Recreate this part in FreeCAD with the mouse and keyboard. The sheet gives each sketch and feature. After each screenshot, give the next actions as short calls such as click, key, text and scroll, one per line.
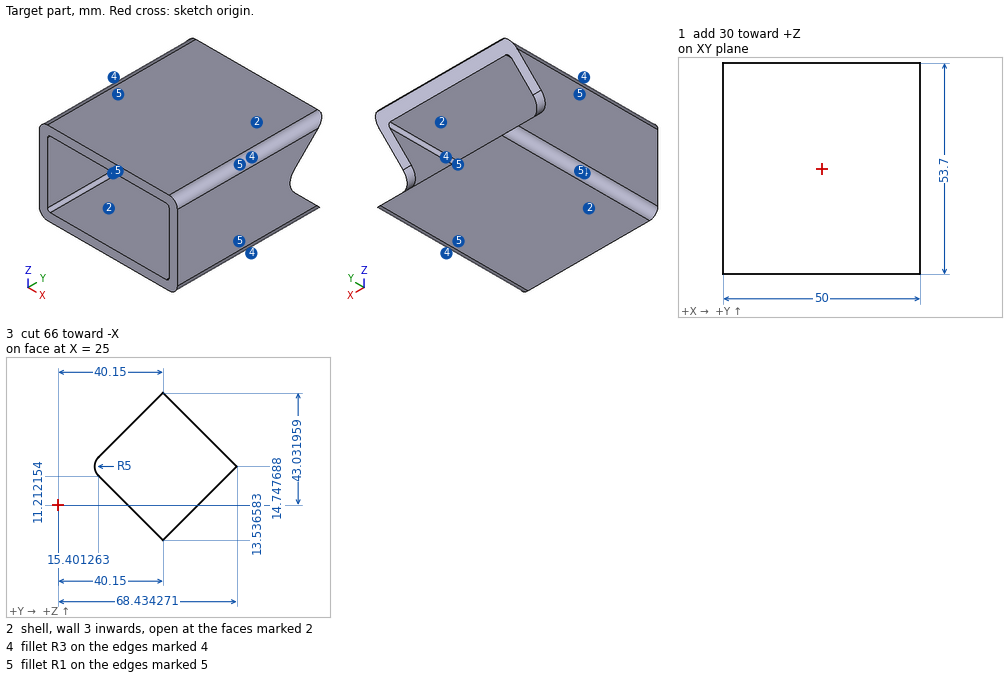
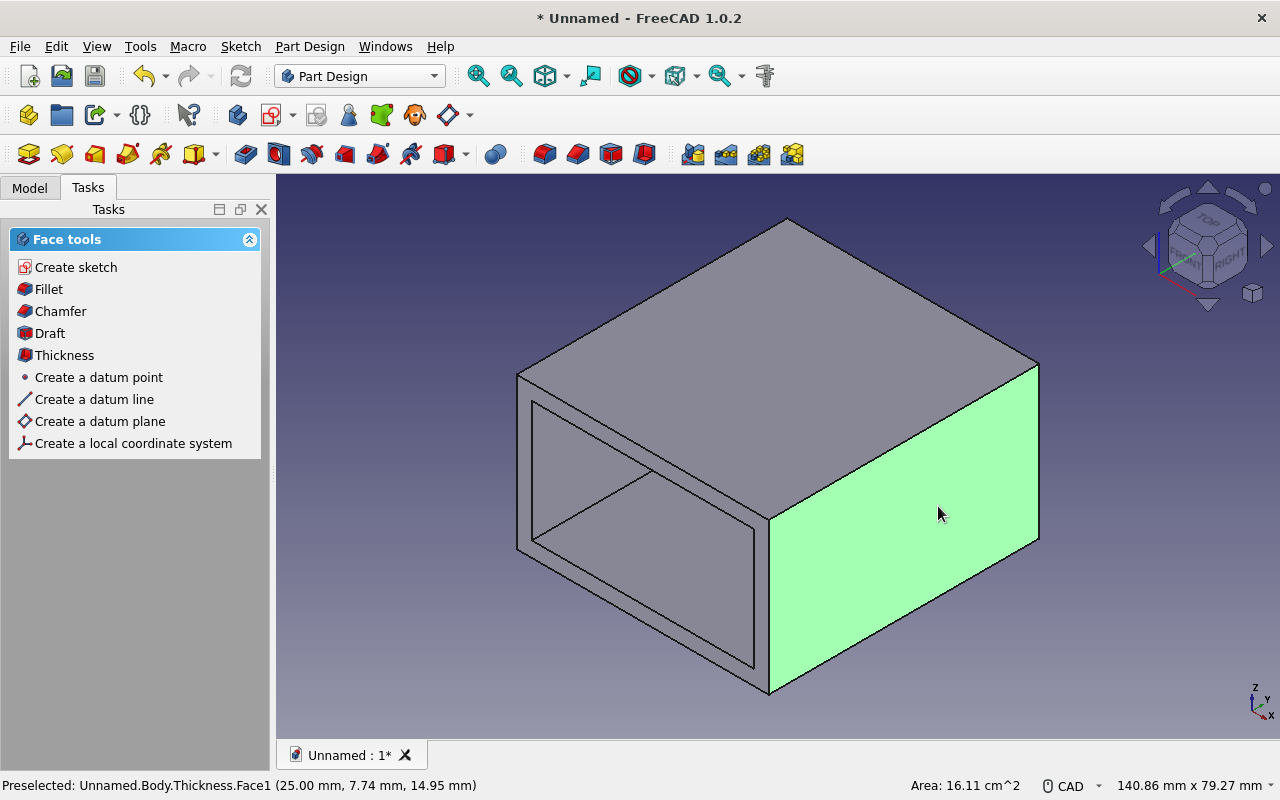
click(270, 116)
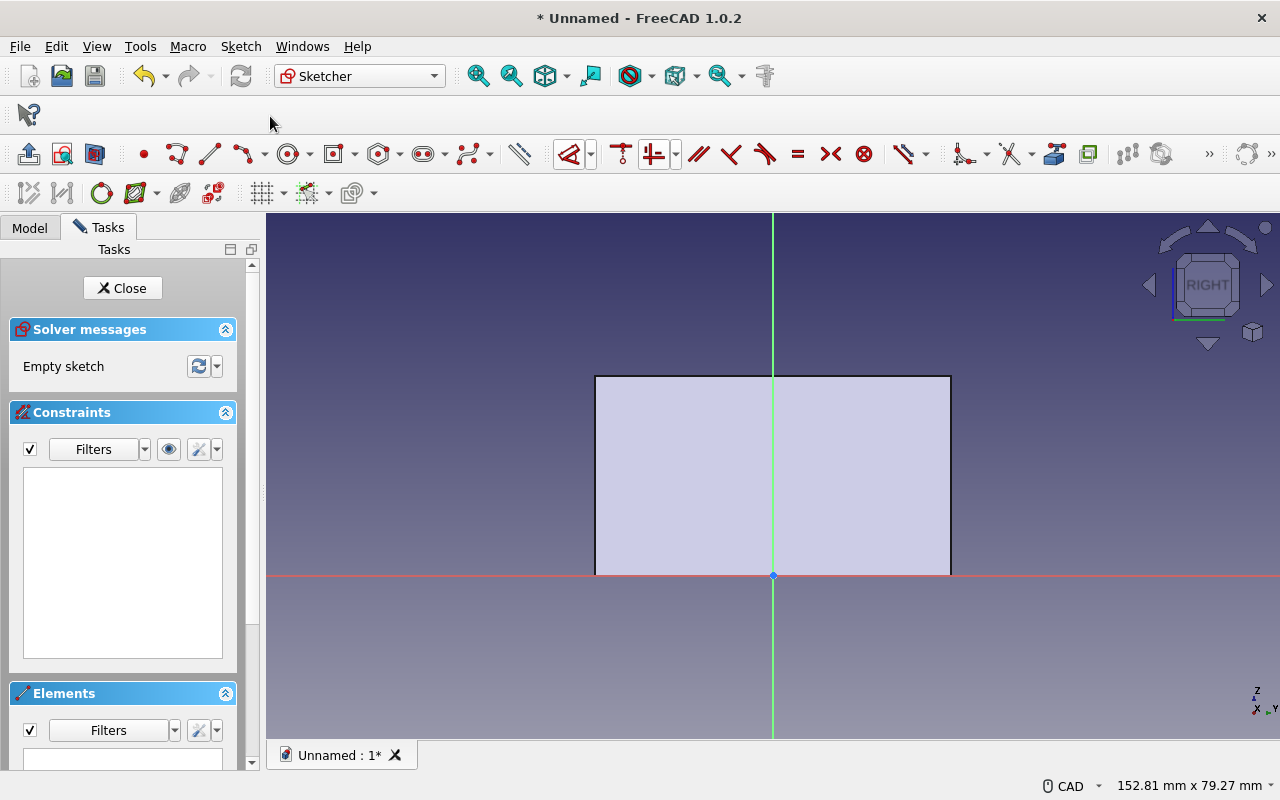
scroll(294, 468, down, 1)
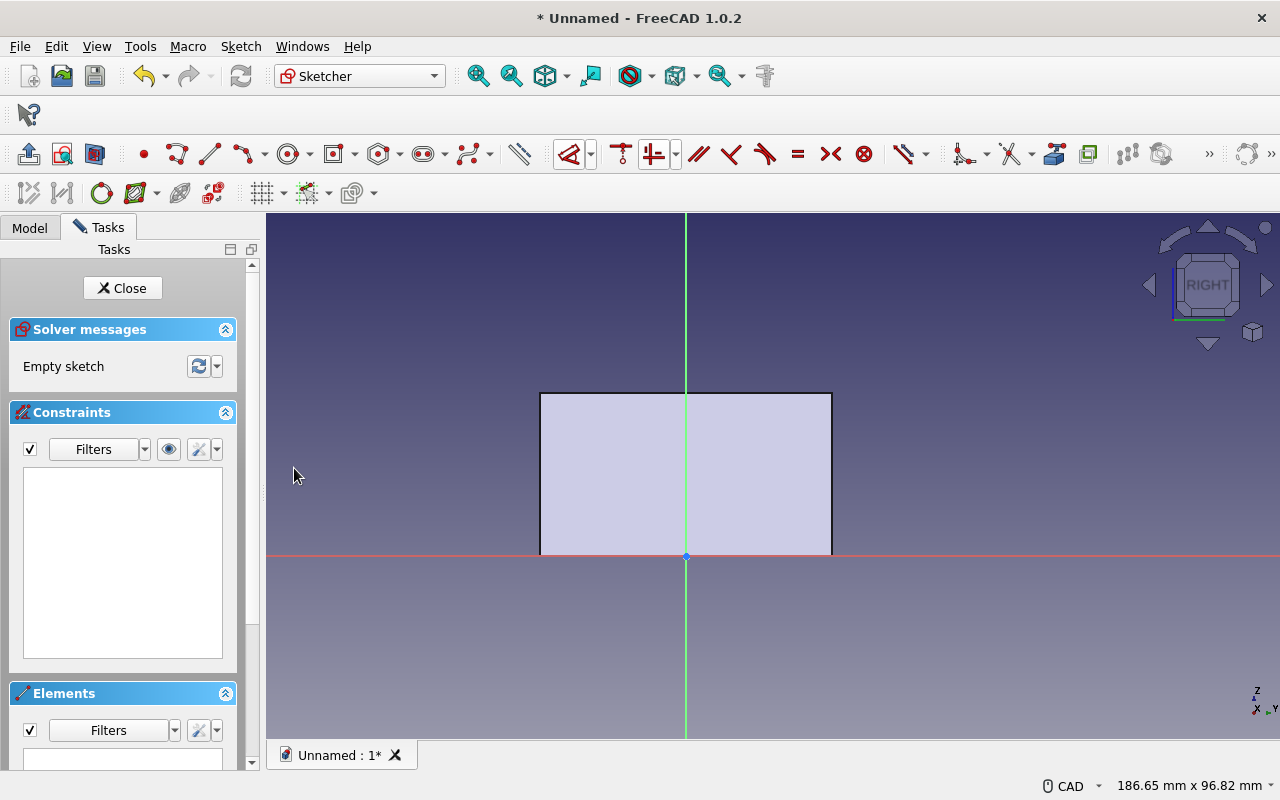
click(177, 154)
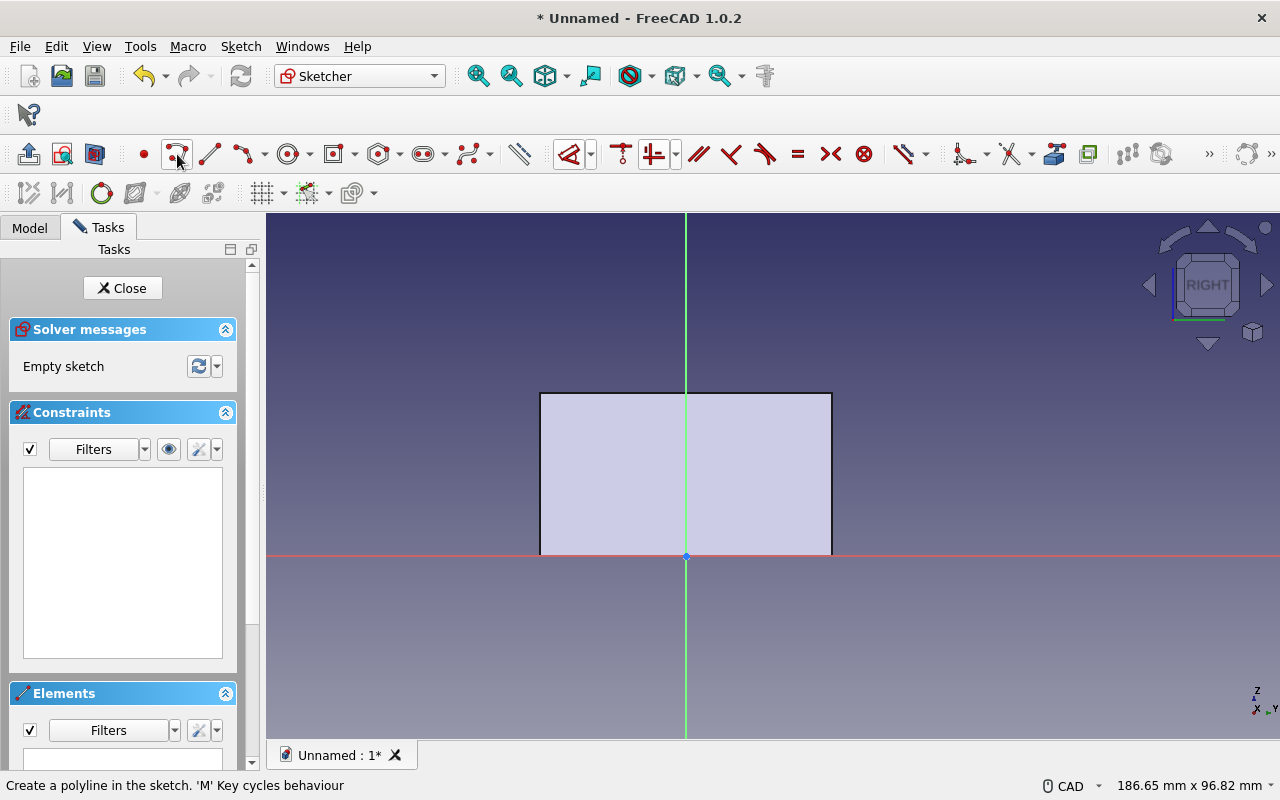
click(770, 495)
click(904, 630)
click(1058, 476)
click(904, 322)
click(770, 457)
right_click(770, 457)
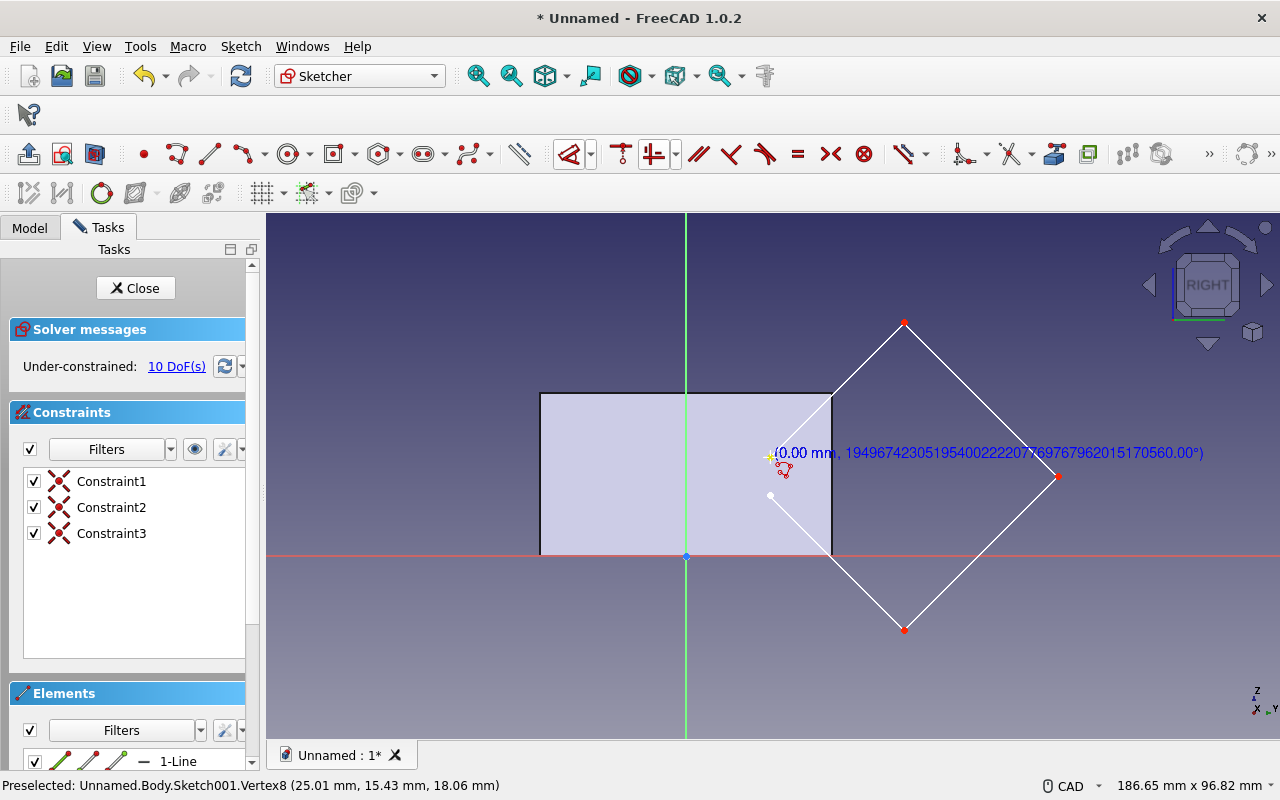
key(g)
key(3)
key(a)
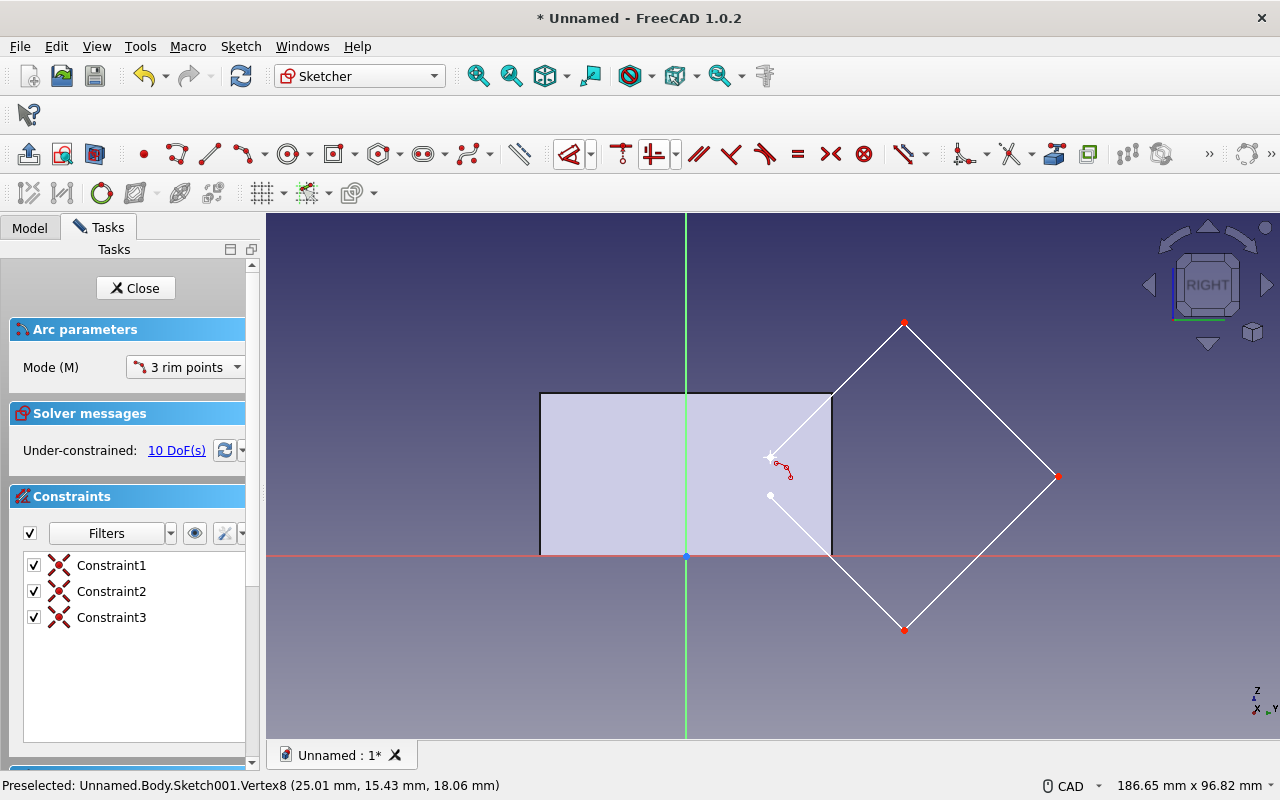
click(770, 458)
click(770, 496)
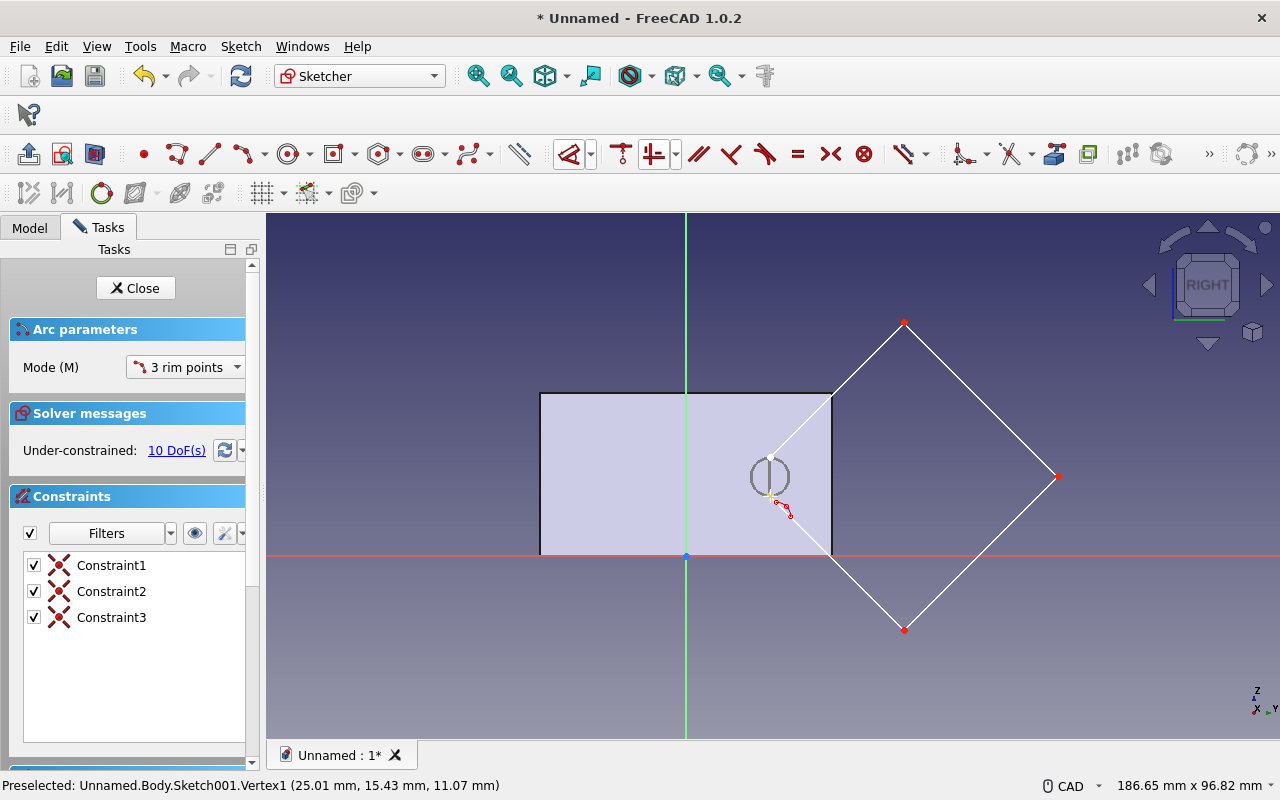
scroll(762, 476, up, 4)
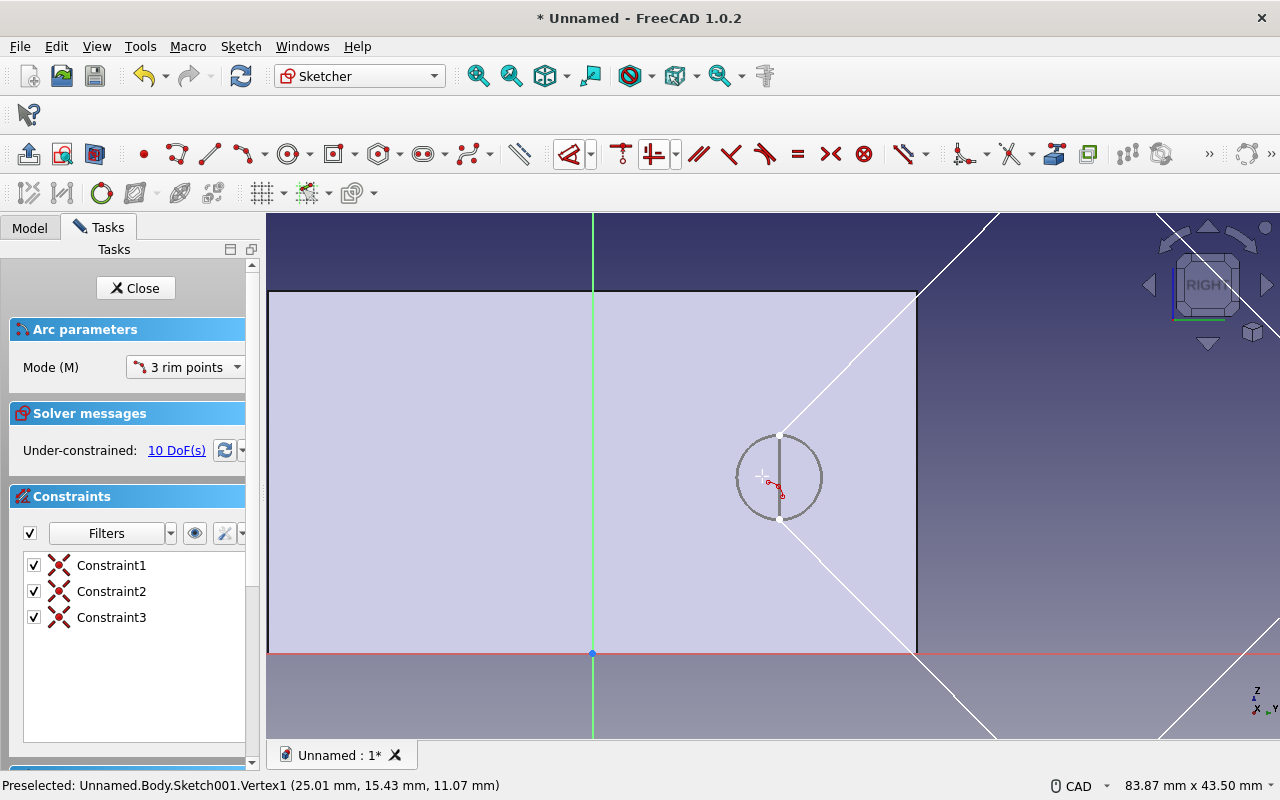
click(761, 475)
key(Escape)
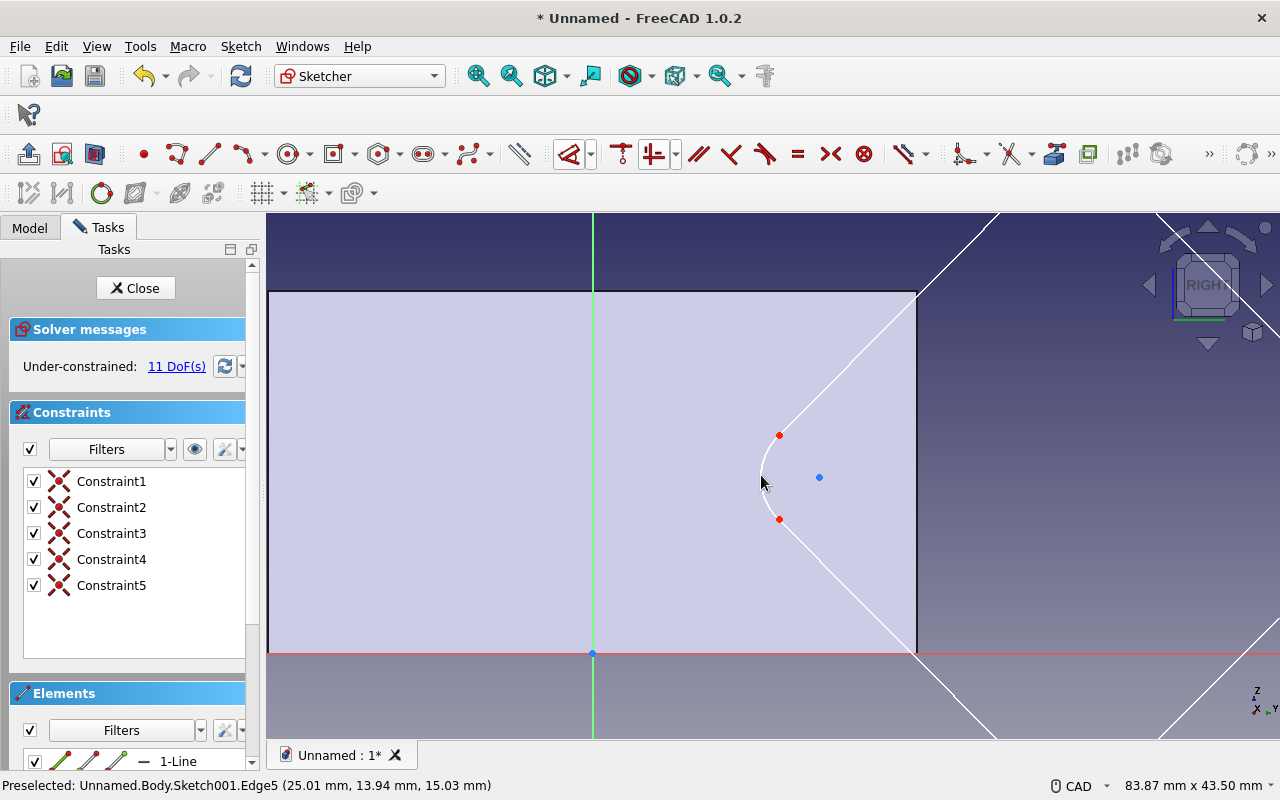
click(869, 610)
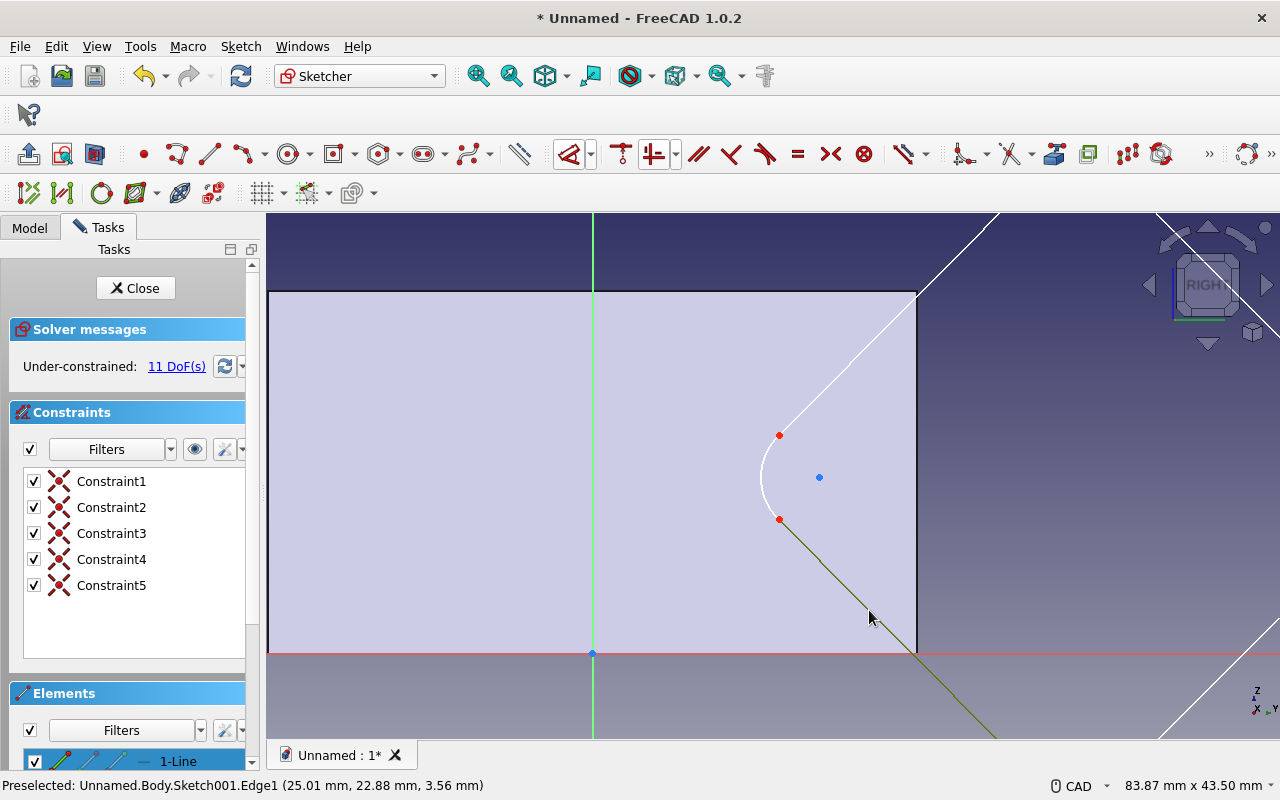
click(764, 459)